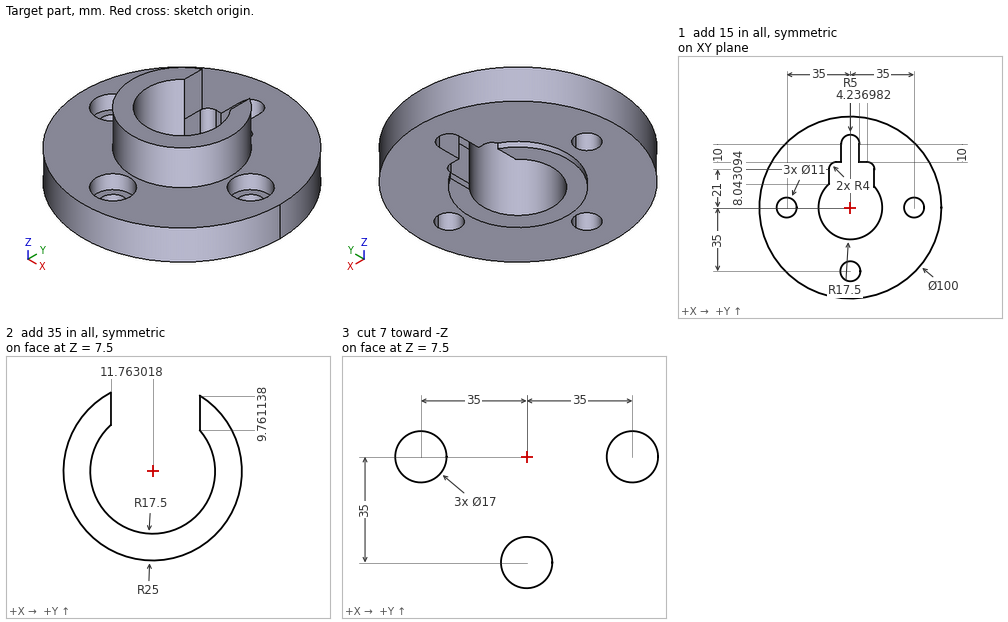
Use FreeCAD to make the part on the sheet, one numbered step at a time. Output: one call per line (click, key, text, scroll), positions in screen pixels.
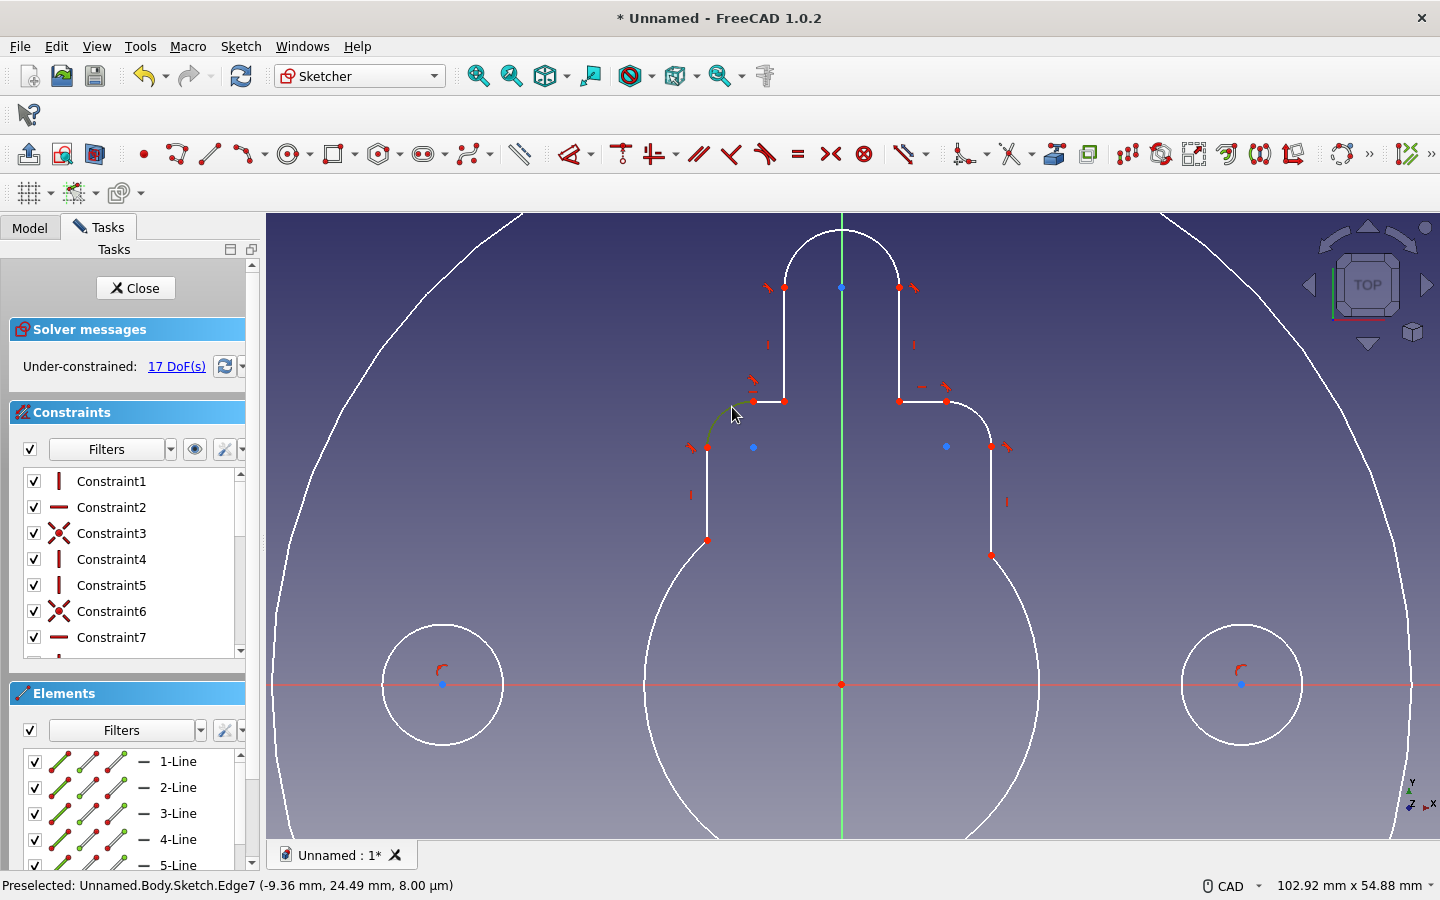
click(987, 426)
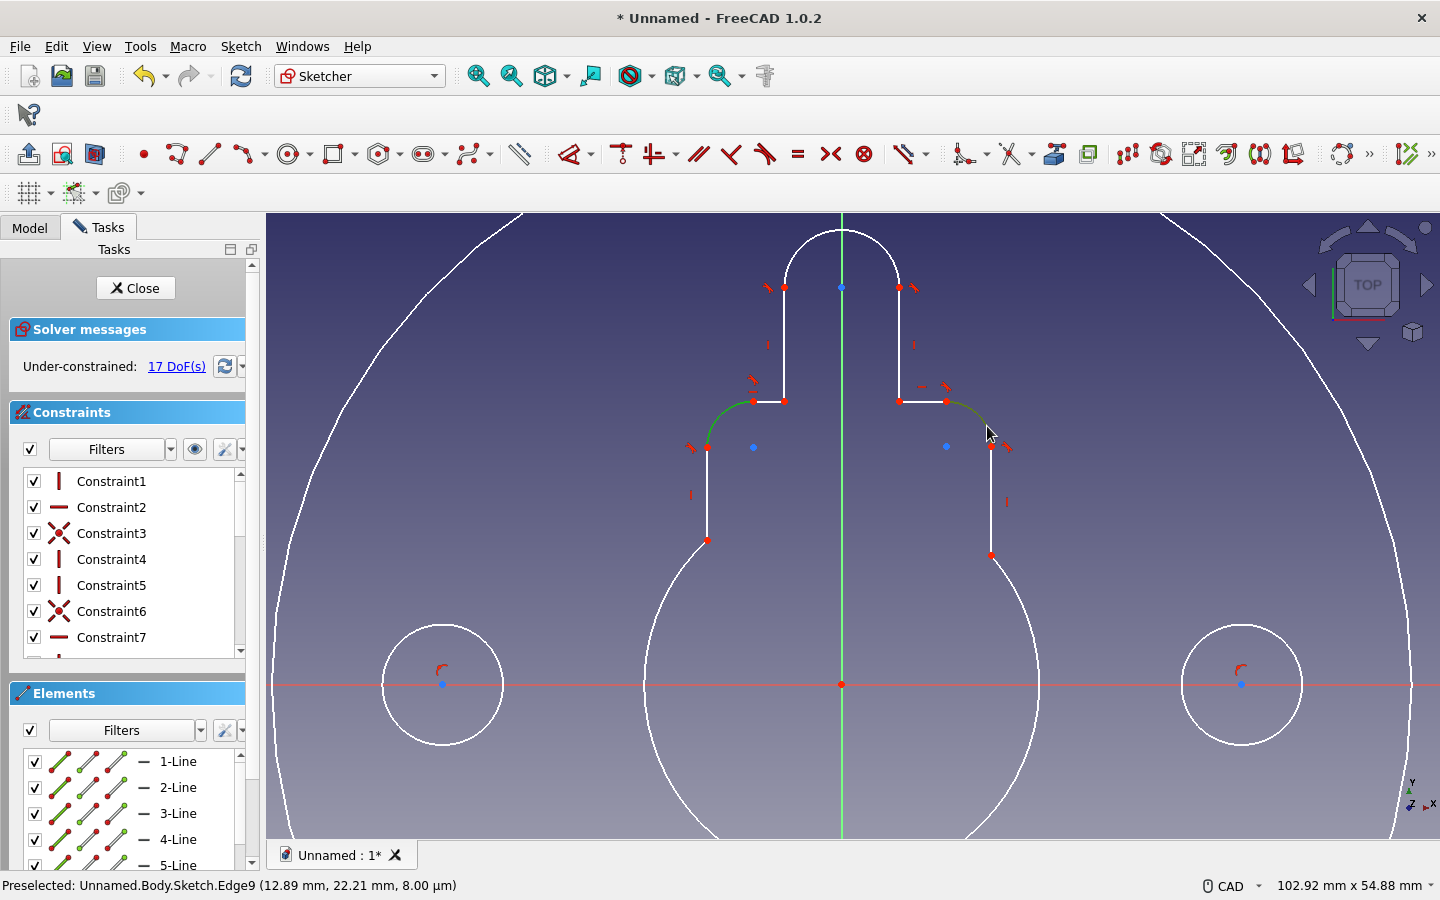
key(e)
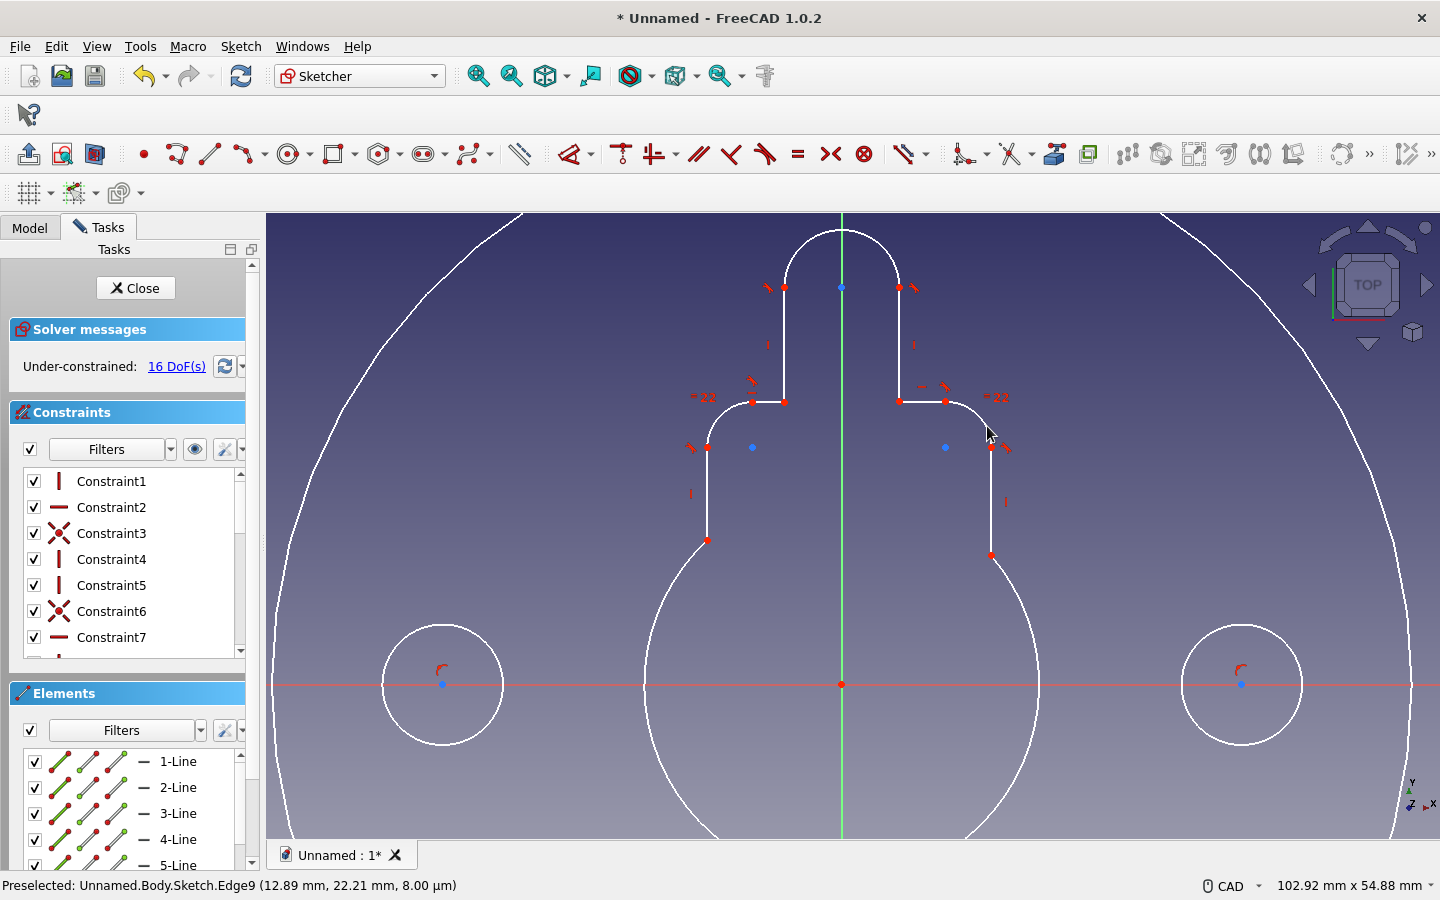
scroll(751, 434, down, 5)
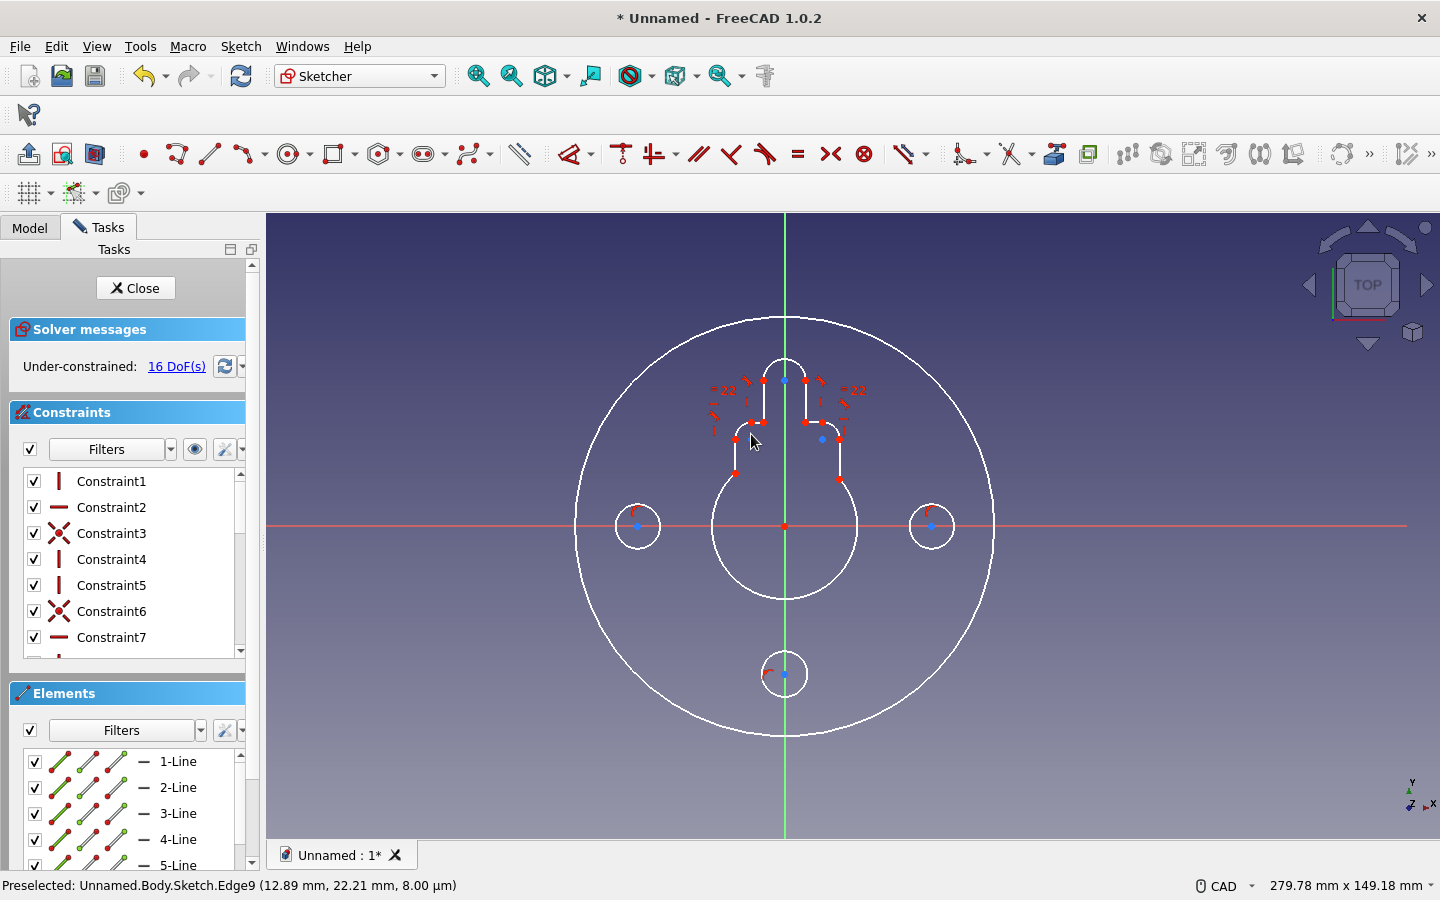
click(801, 658)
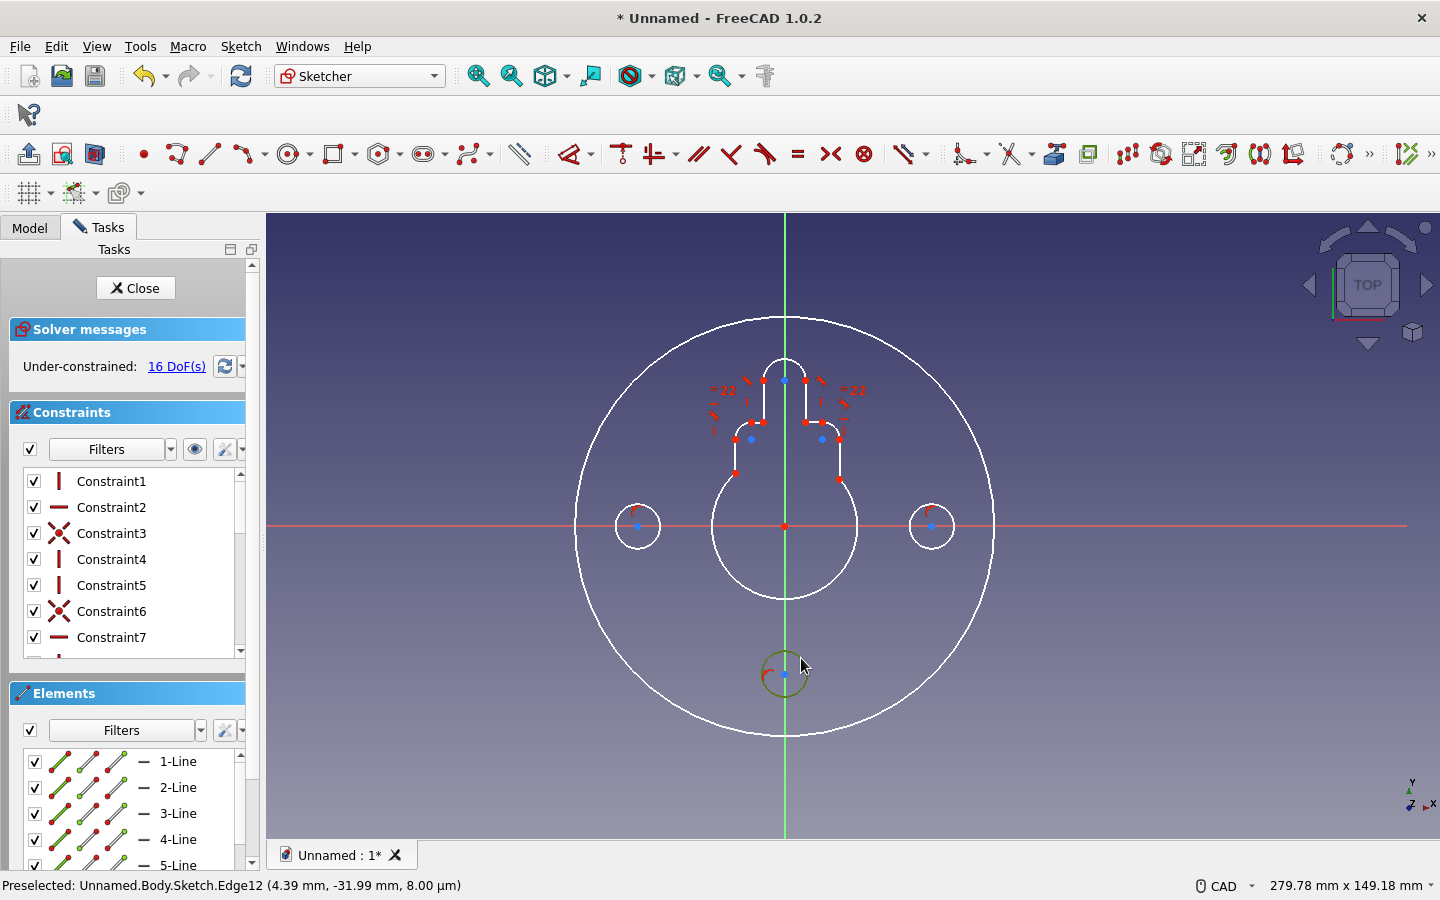
click(653, 511)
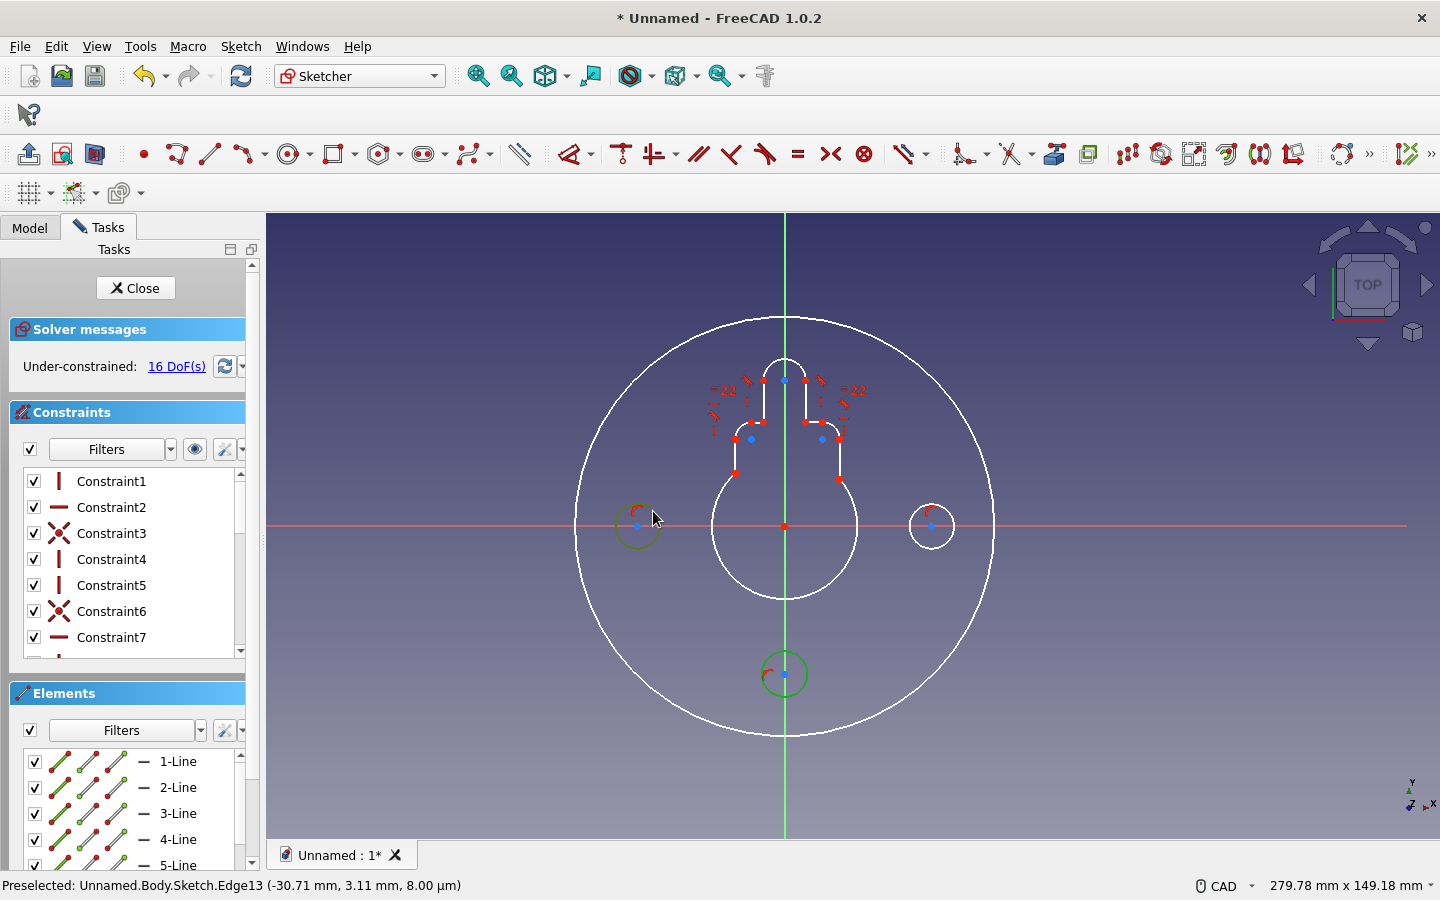
click(947, 511)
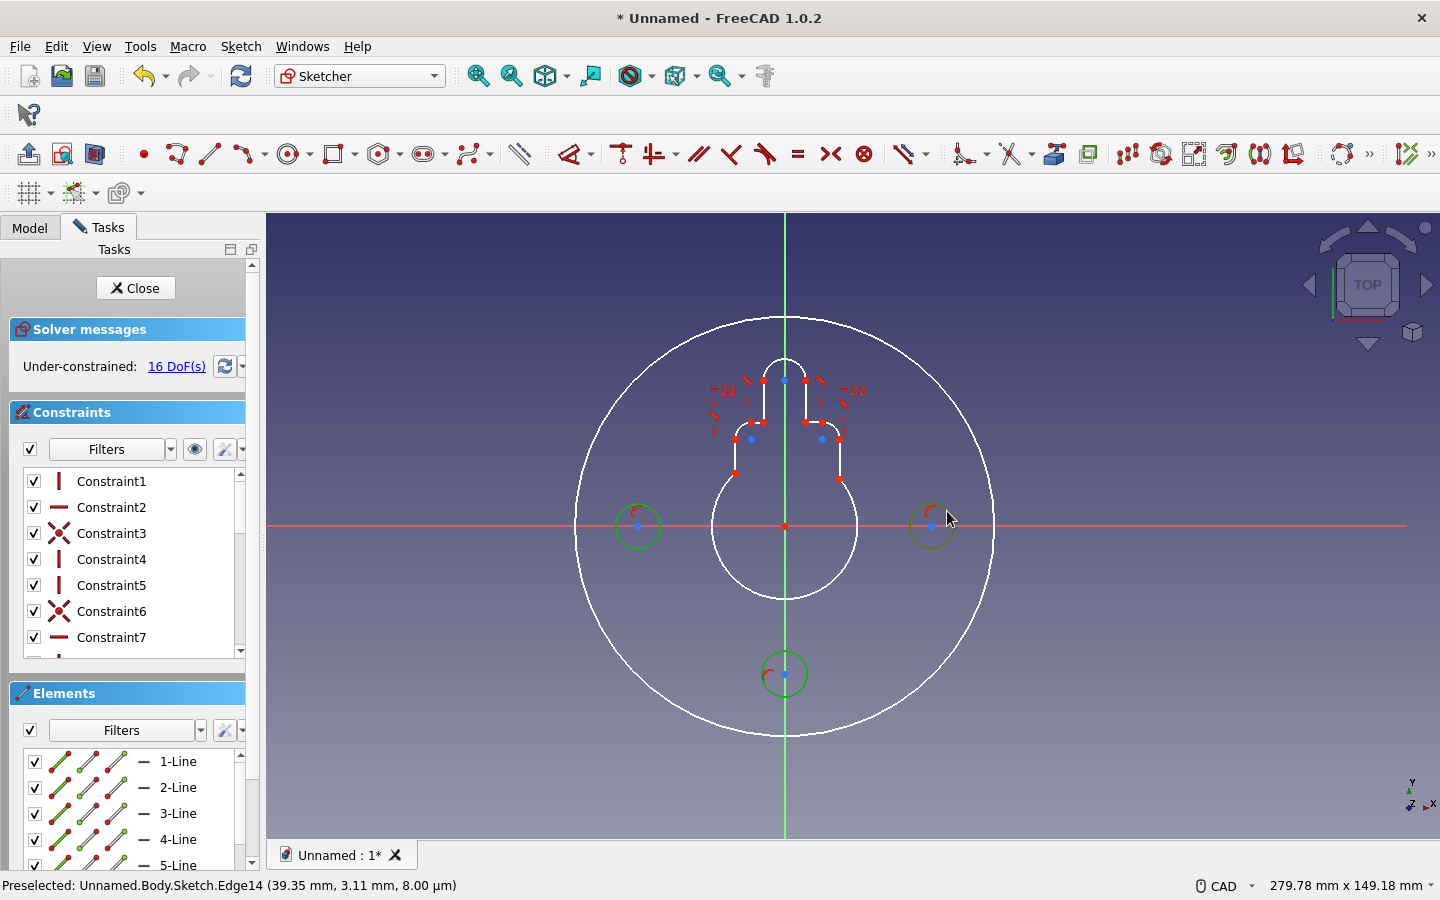
key(e)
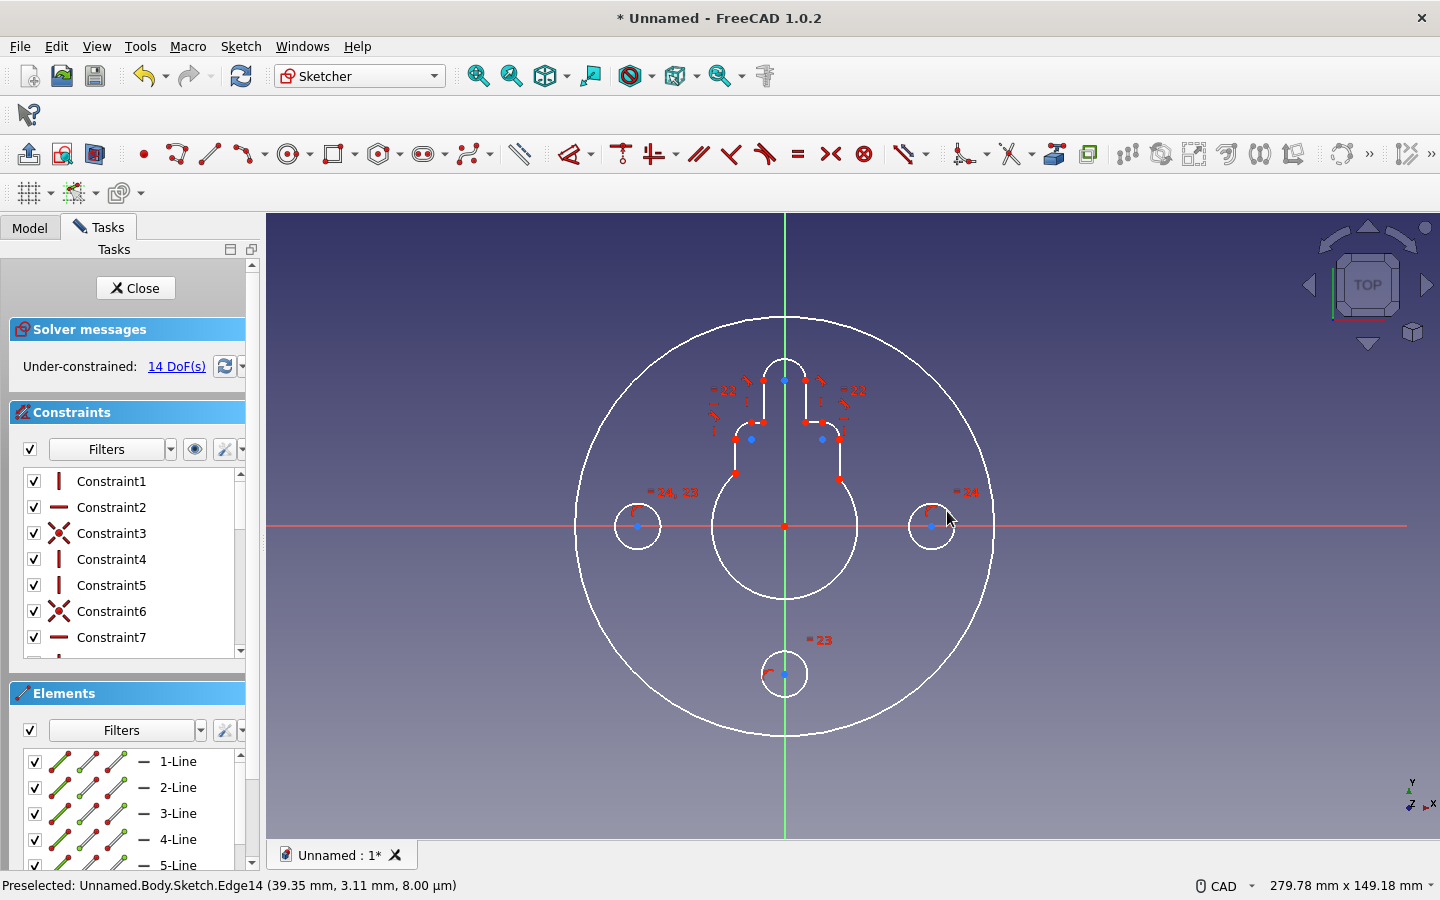
click(785, 380)